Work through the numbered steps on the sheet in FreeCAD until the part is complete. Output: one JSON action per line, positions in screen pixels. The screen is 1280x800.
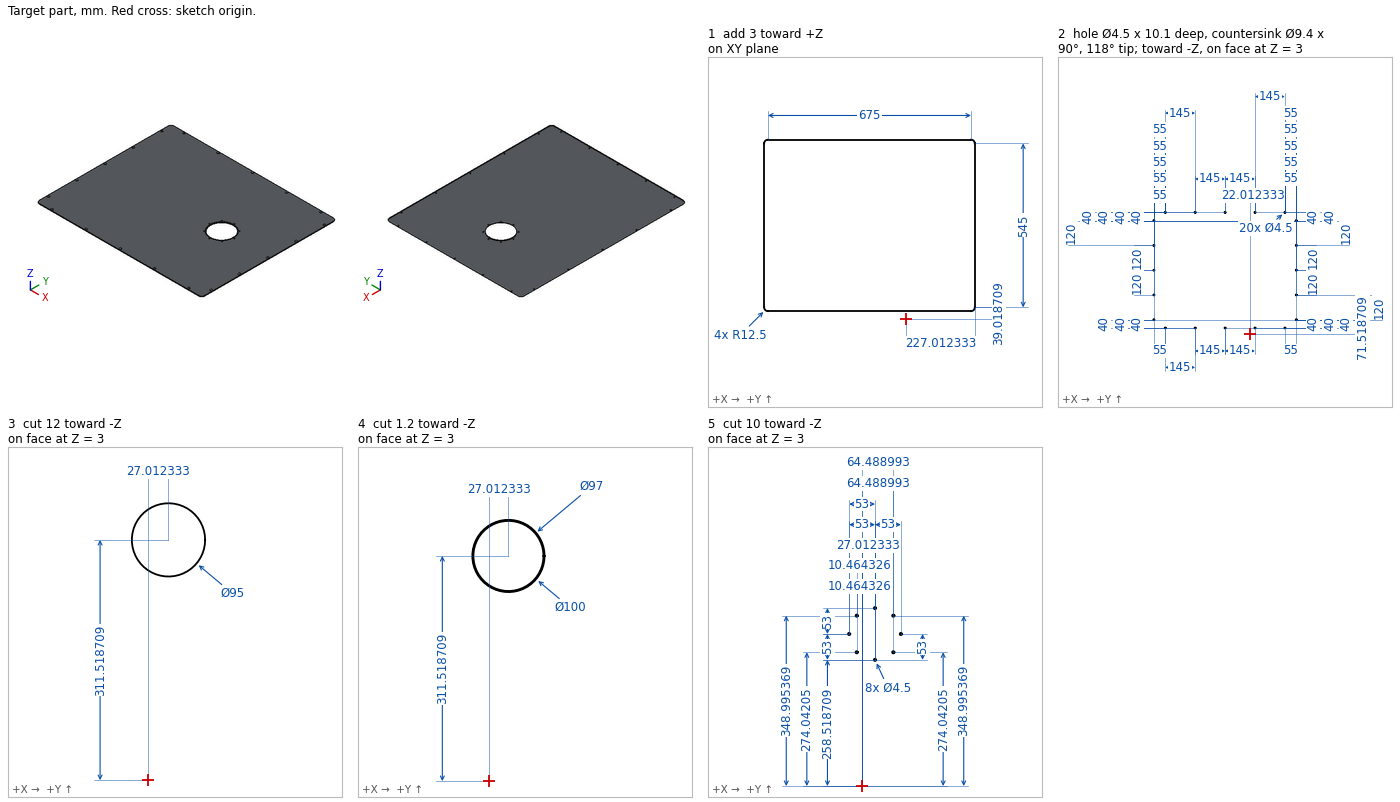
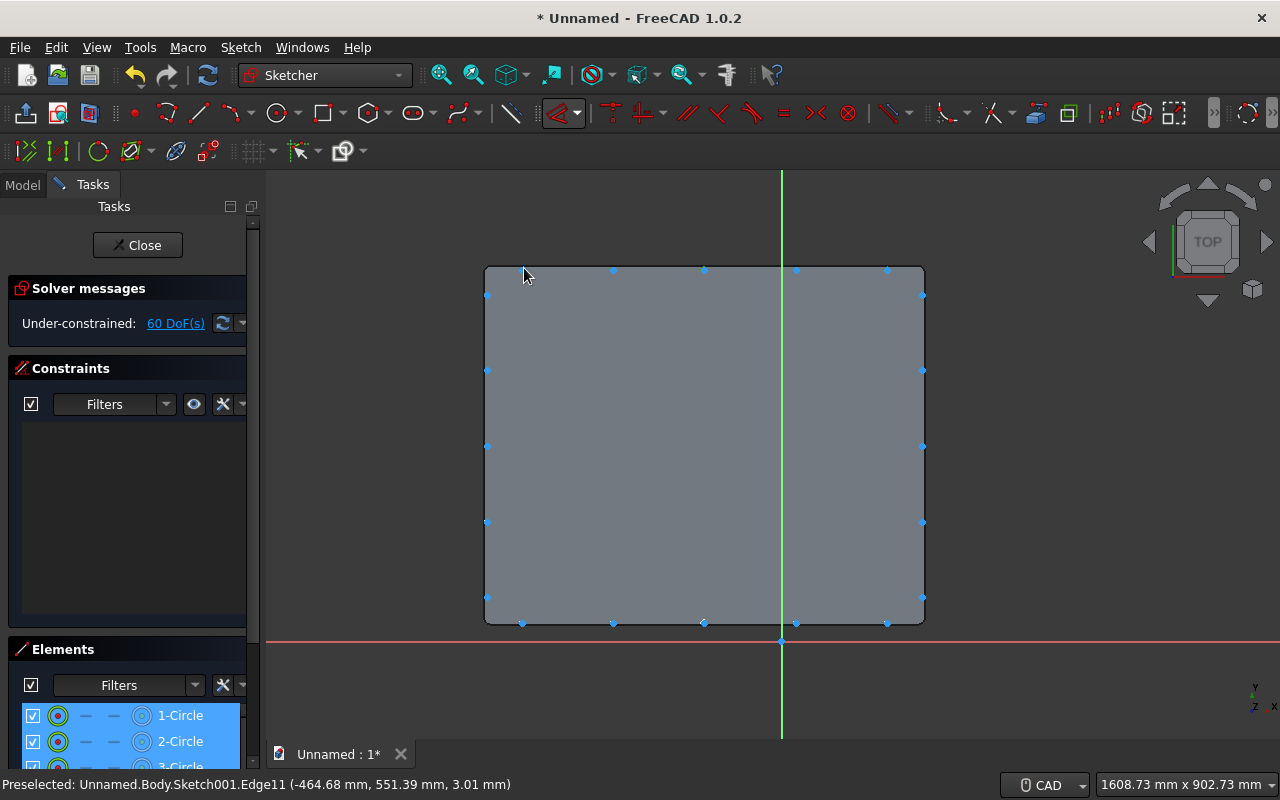
{"action": "scroll", "coordinate": [488, 369], "scroll_direction": "up", "scroll_amount": 11}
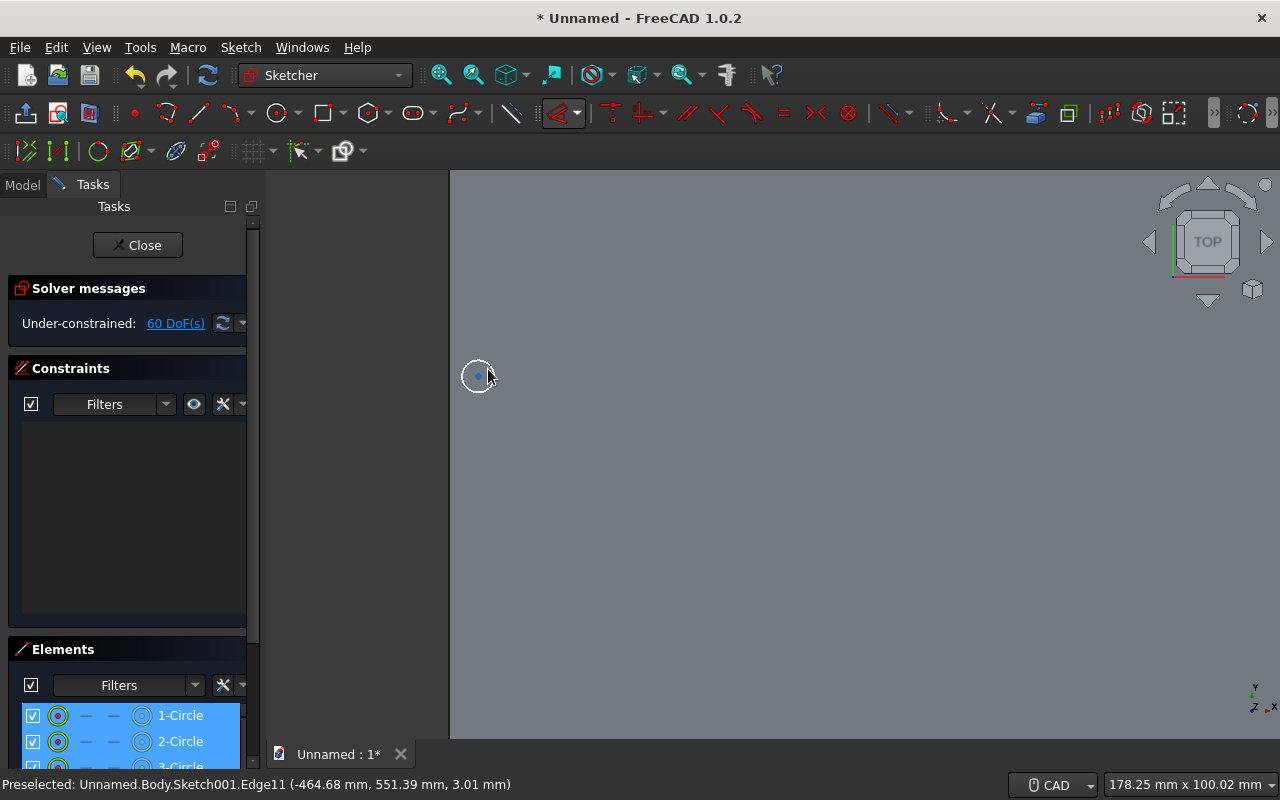
{"action": "left_click", "coordinate": [489, 365]}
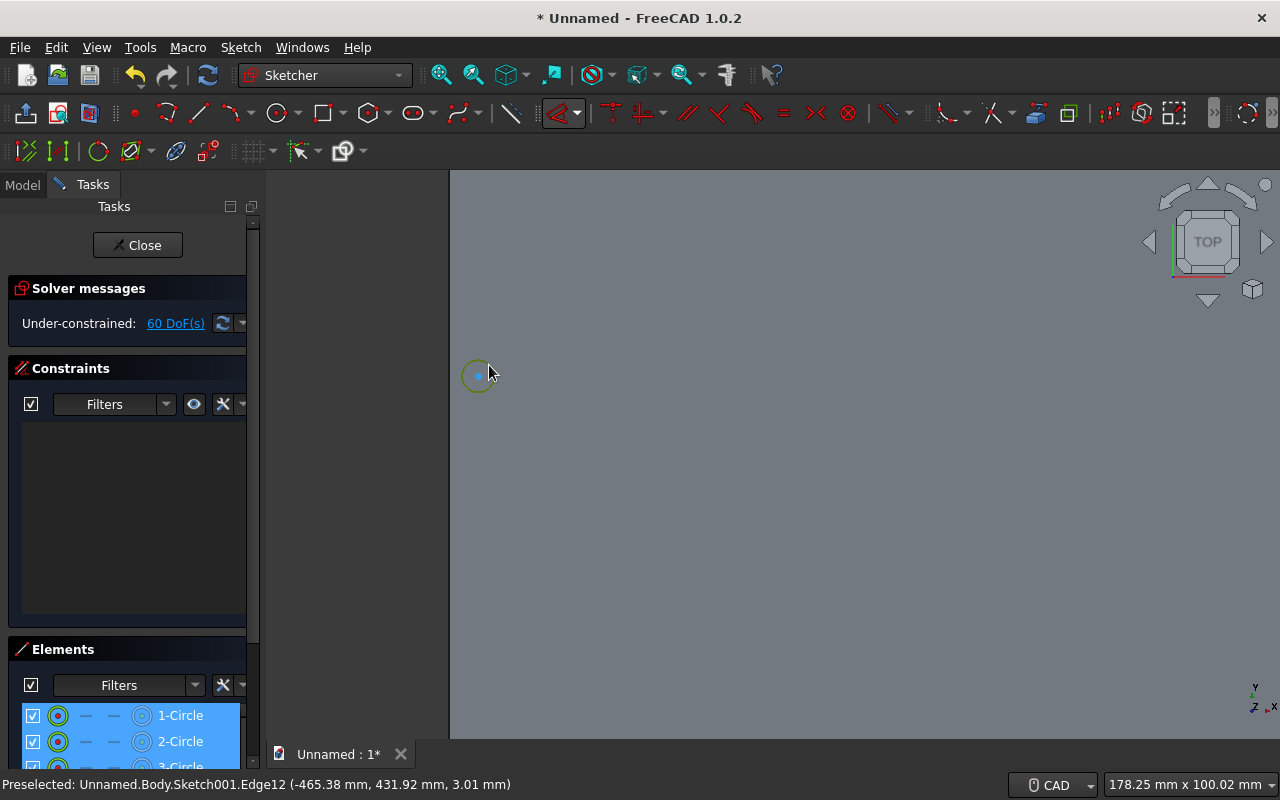
{"action": "scroll", "coordinate": [488, 369], "scroll_direction": "down", "scroll_amount": 11}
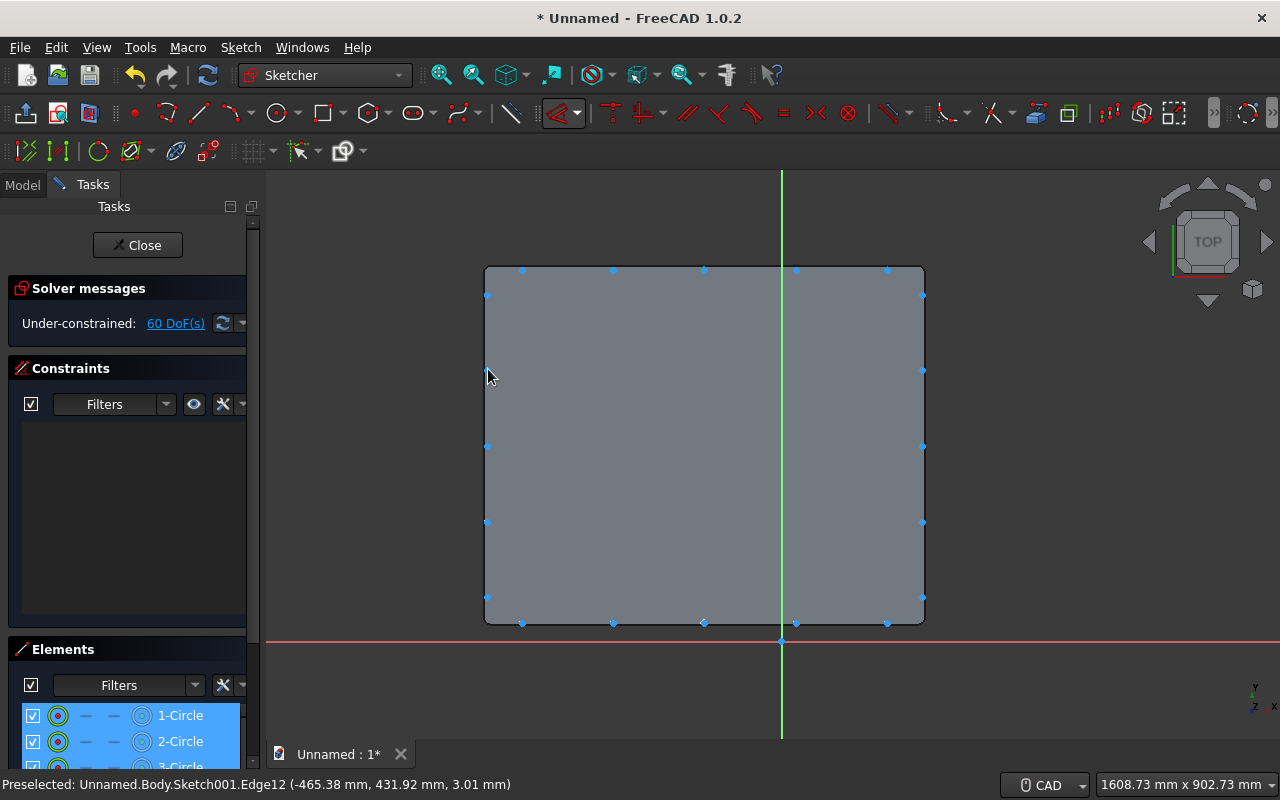
{"action": "scroll", "coordinate": [489, 445], "scroll_direction": "up", "scroll_amount": 10}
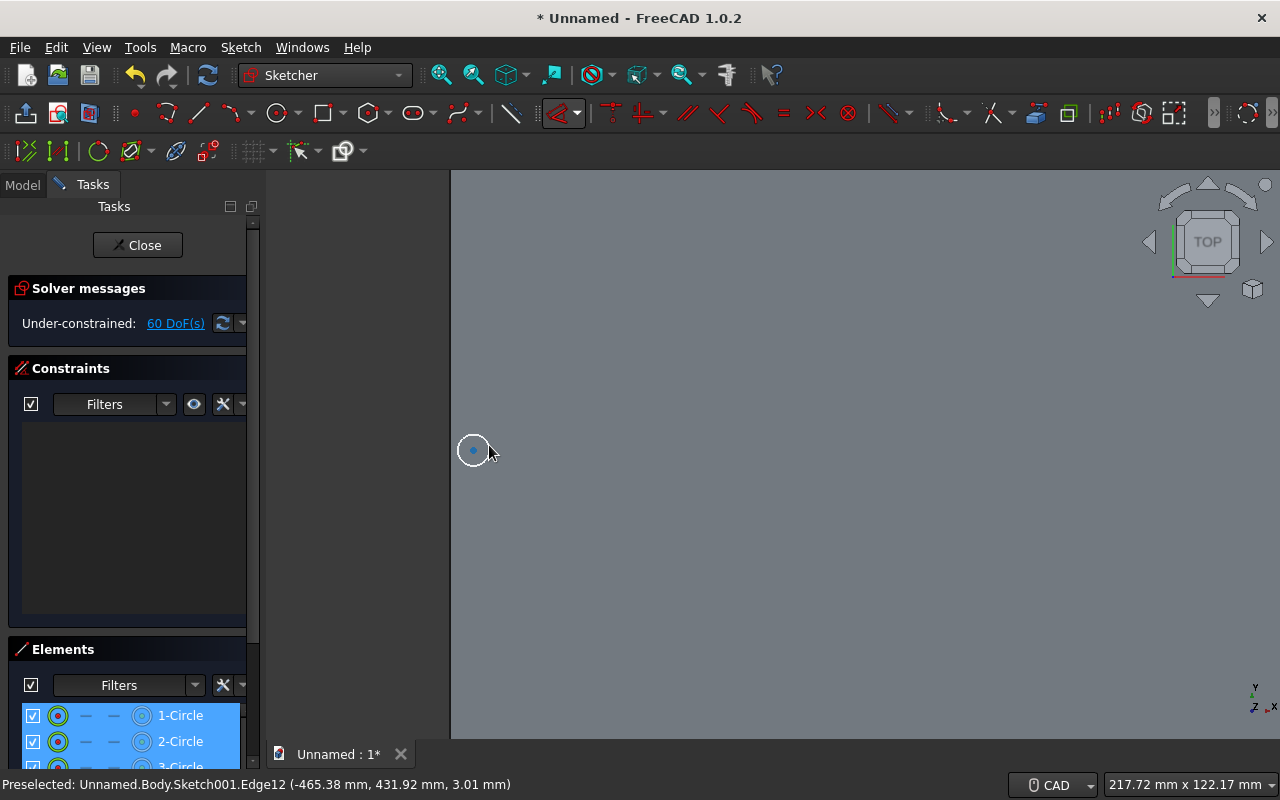
{"action": "left_click", "coordinate": [485, 439]}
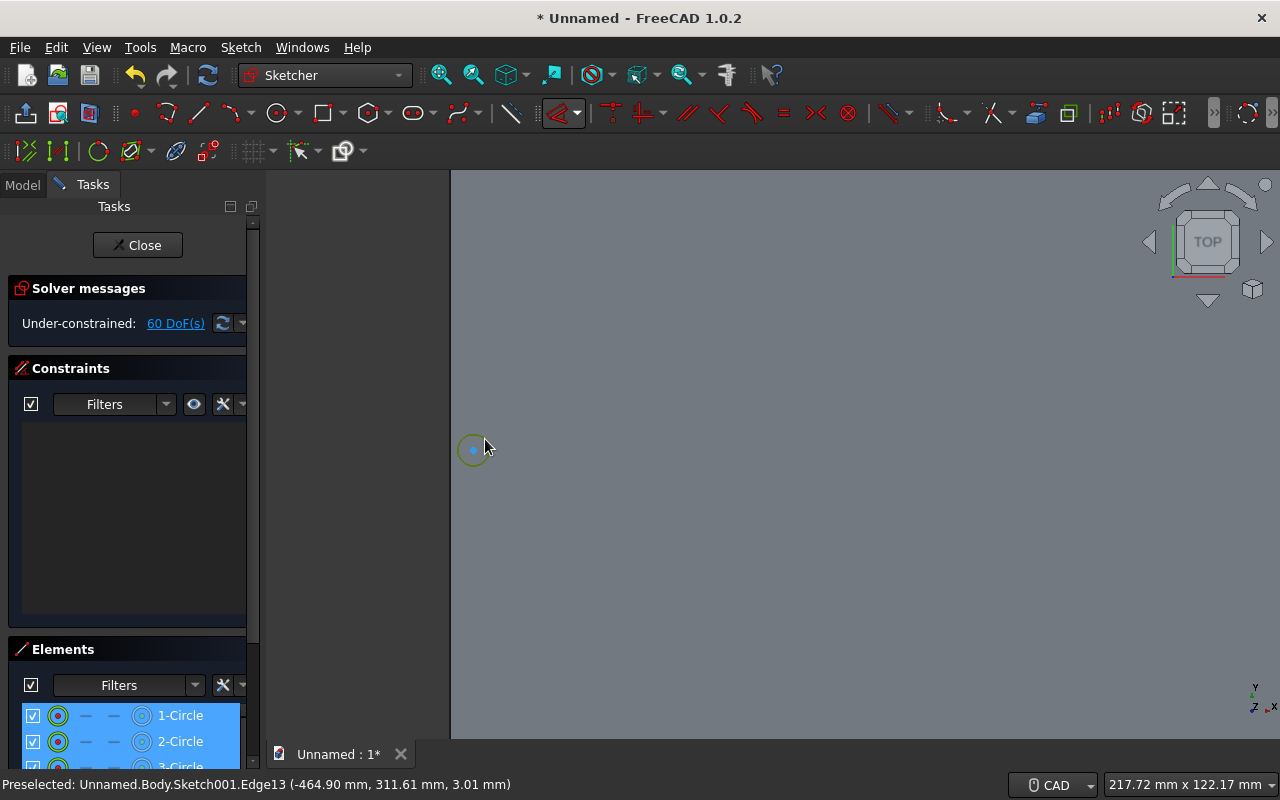
{"action": "scroll", "coordinate": [489, 446], "scroll_direction": "down", "scroll_amount": 10}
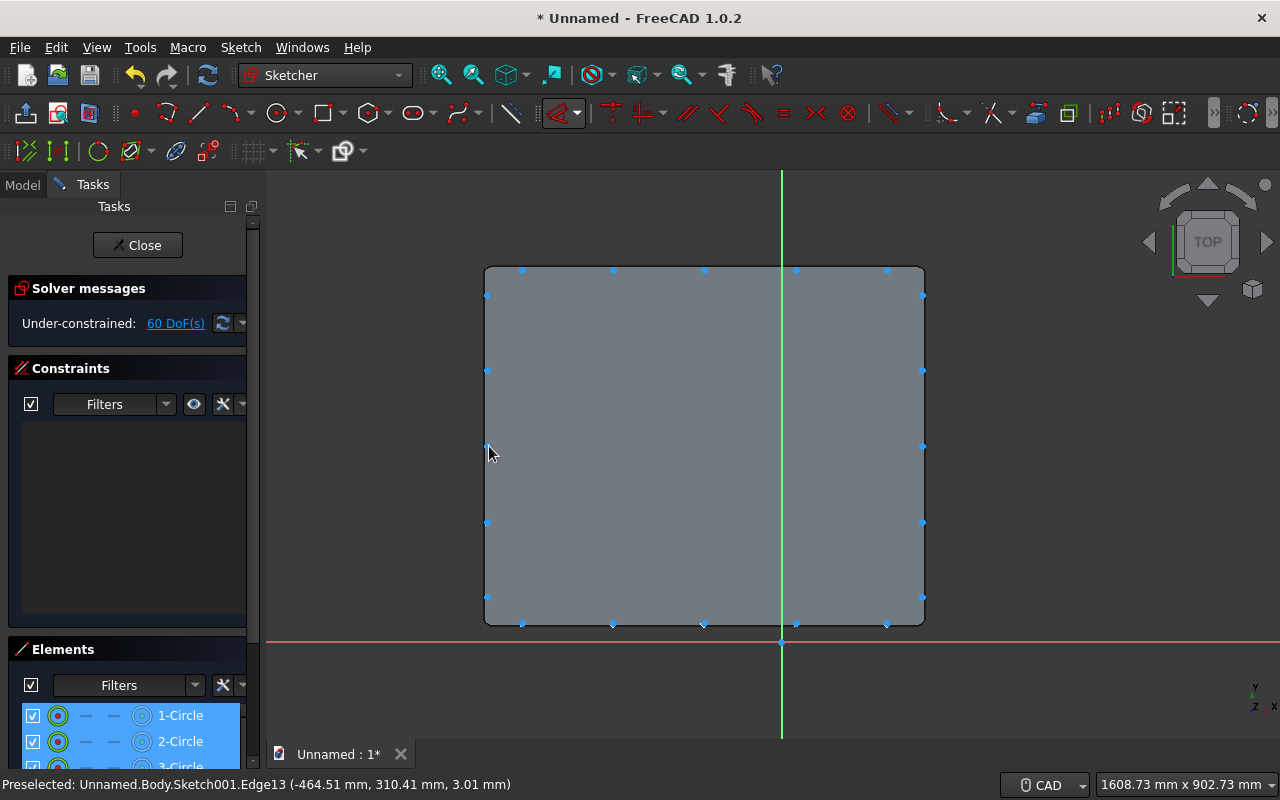
{"action": "scroll", "coordinate": [489, 521], "scroll_direction": "up", "scroll_amount": 9}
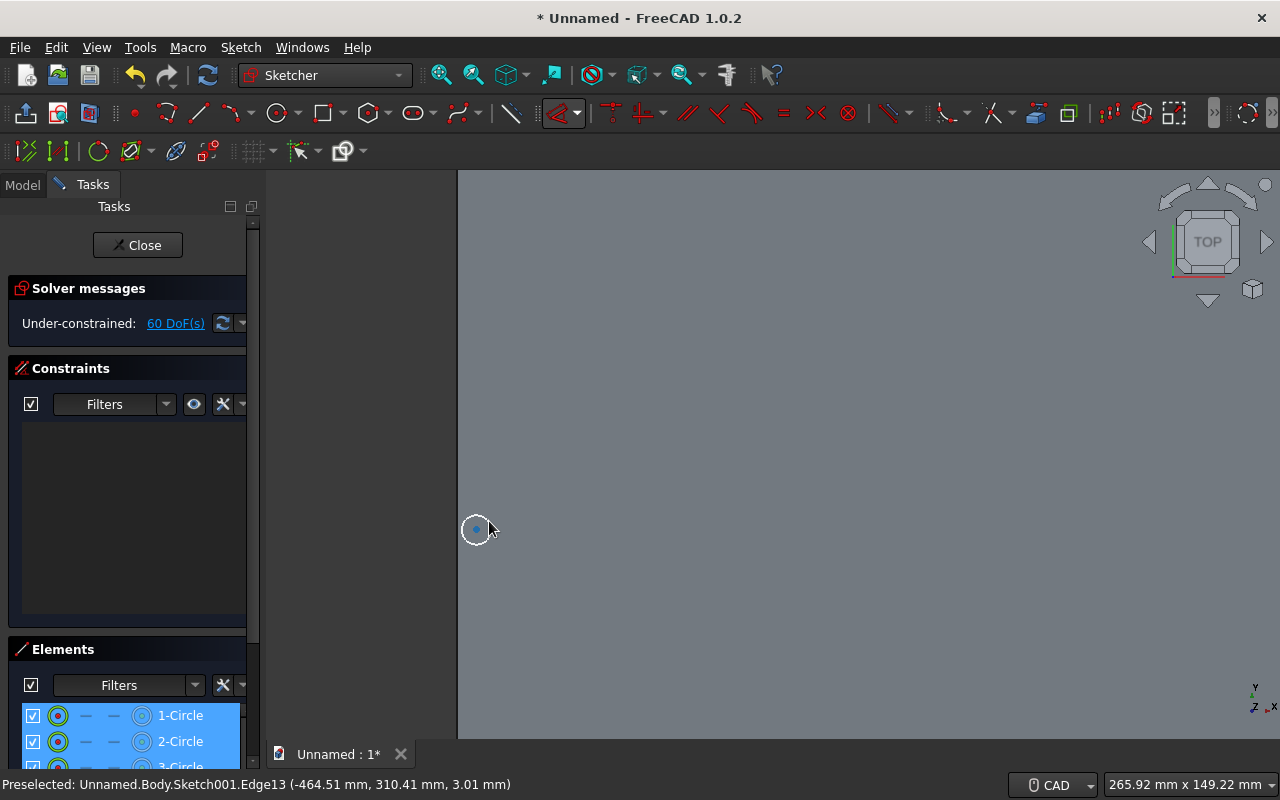
{"action": "left_click", "coordinate": [487, 520]}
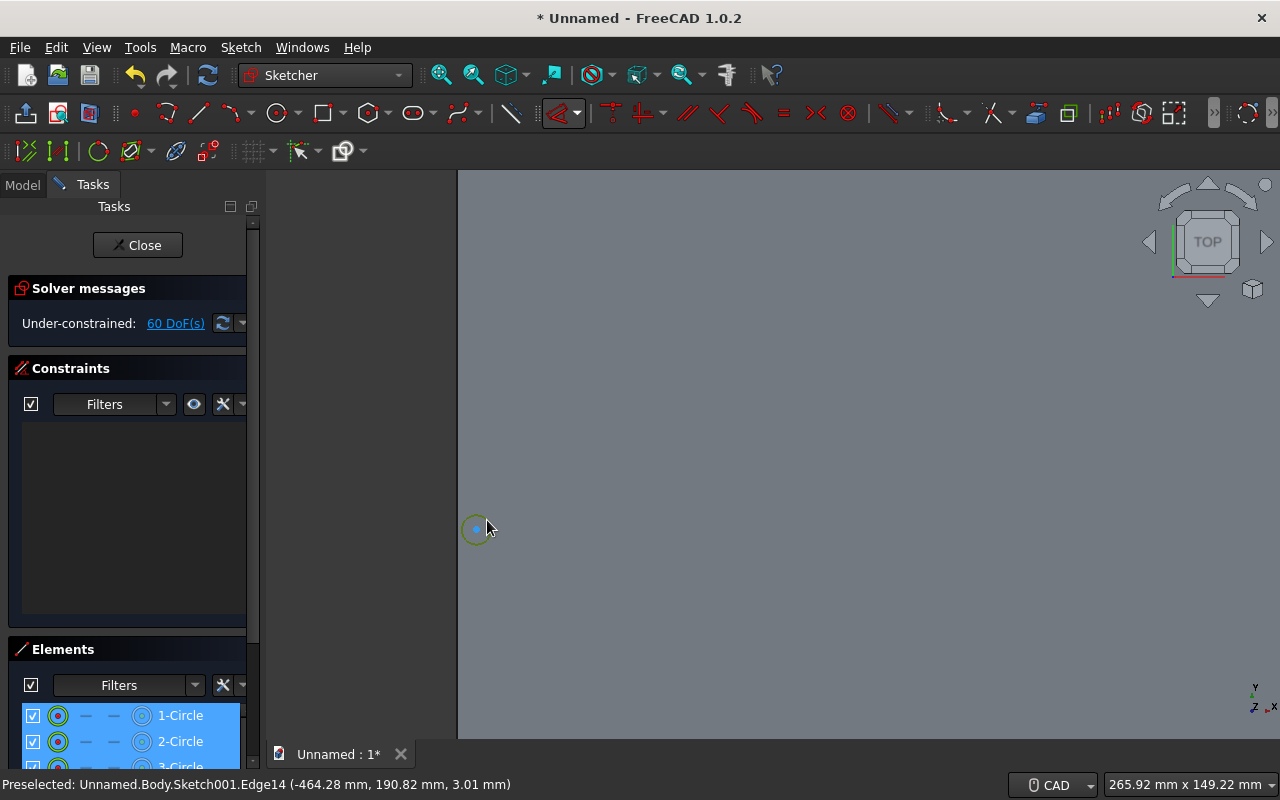
{"action": "scroll", "coordinate": [489, 521], "scroll_direction": "down", "scroll_amount": 9}